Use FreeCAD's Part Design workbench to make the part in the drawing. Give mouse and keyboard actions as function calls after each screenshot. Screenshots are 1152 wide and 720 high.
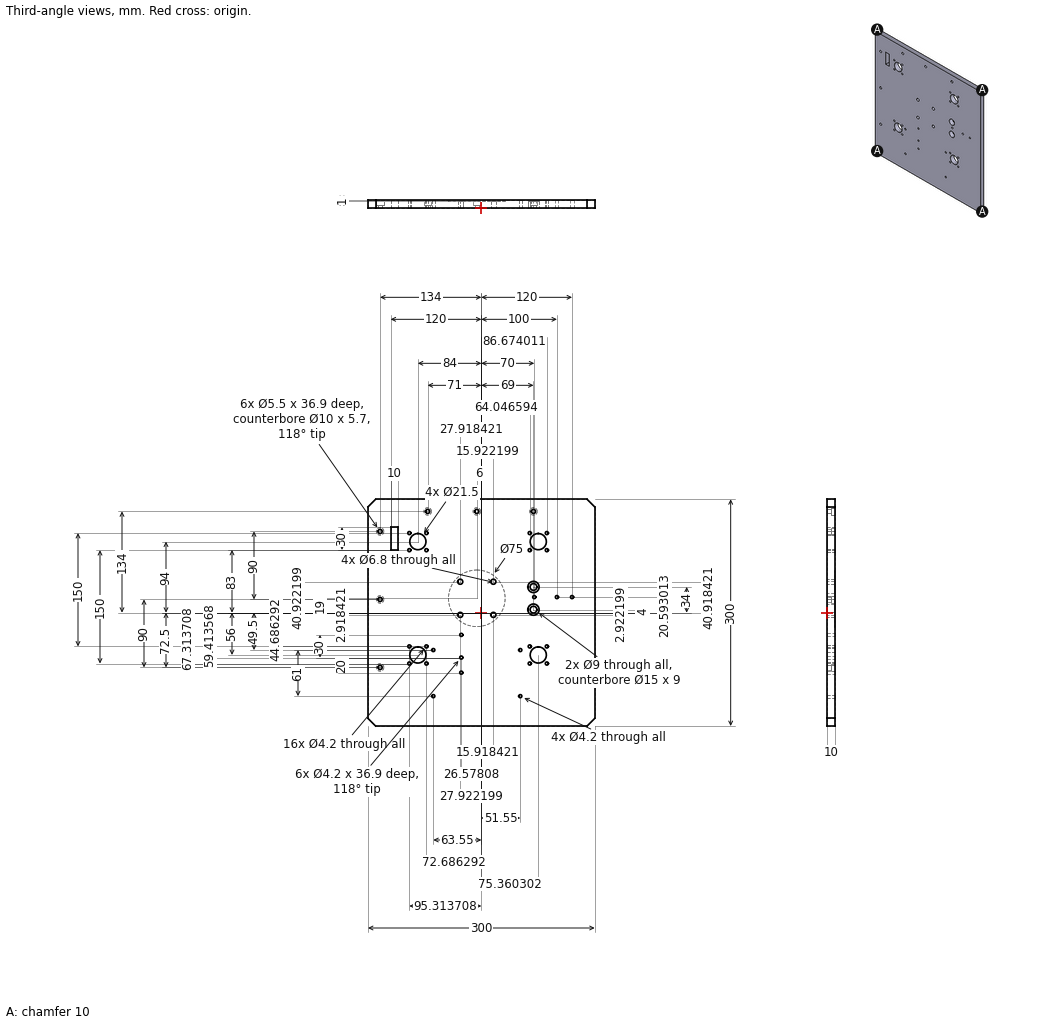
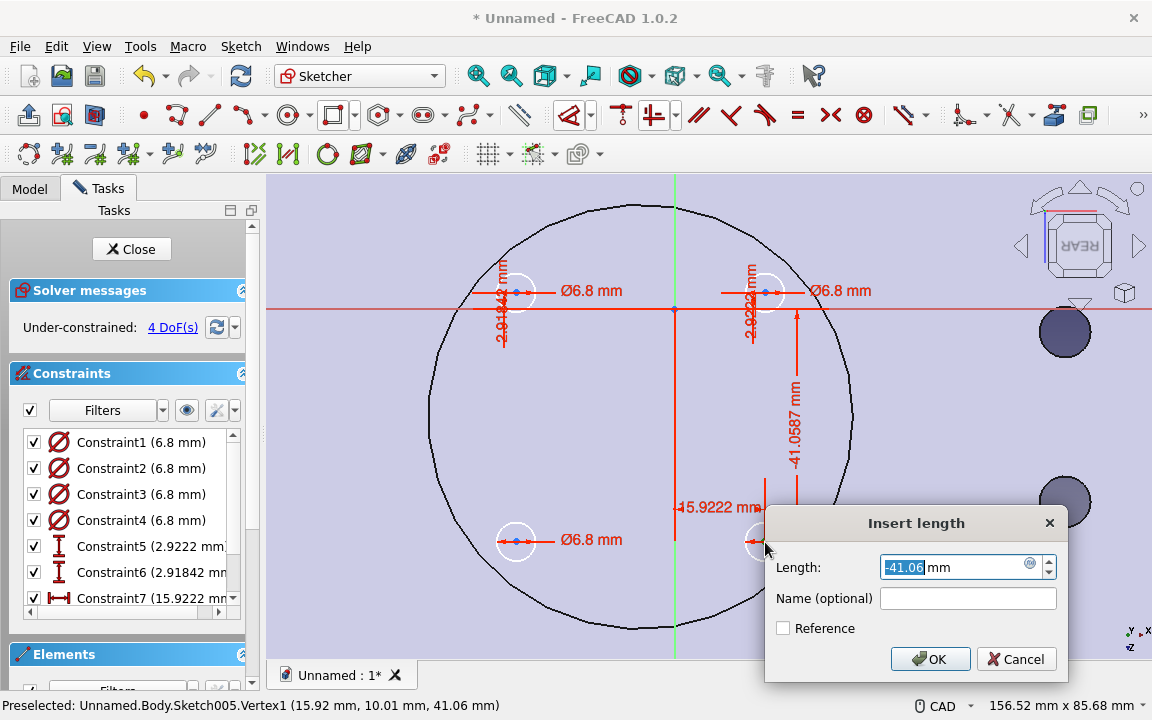
text(-40.918421)
key(Return)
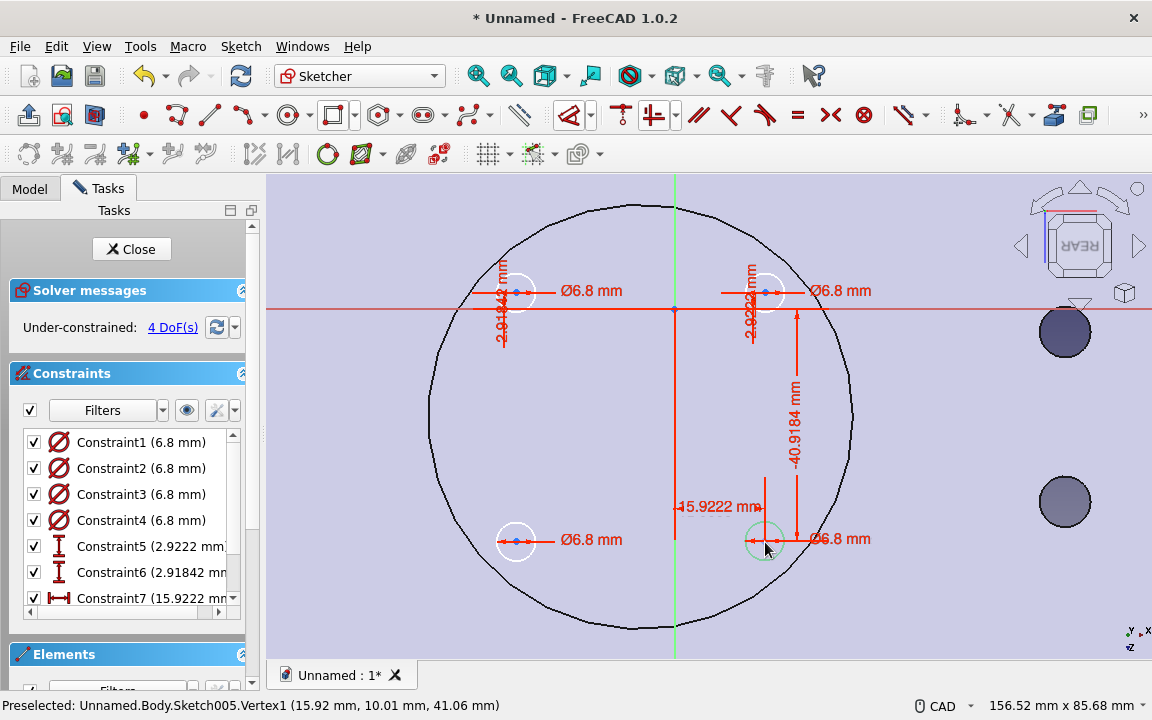
click(765, 293)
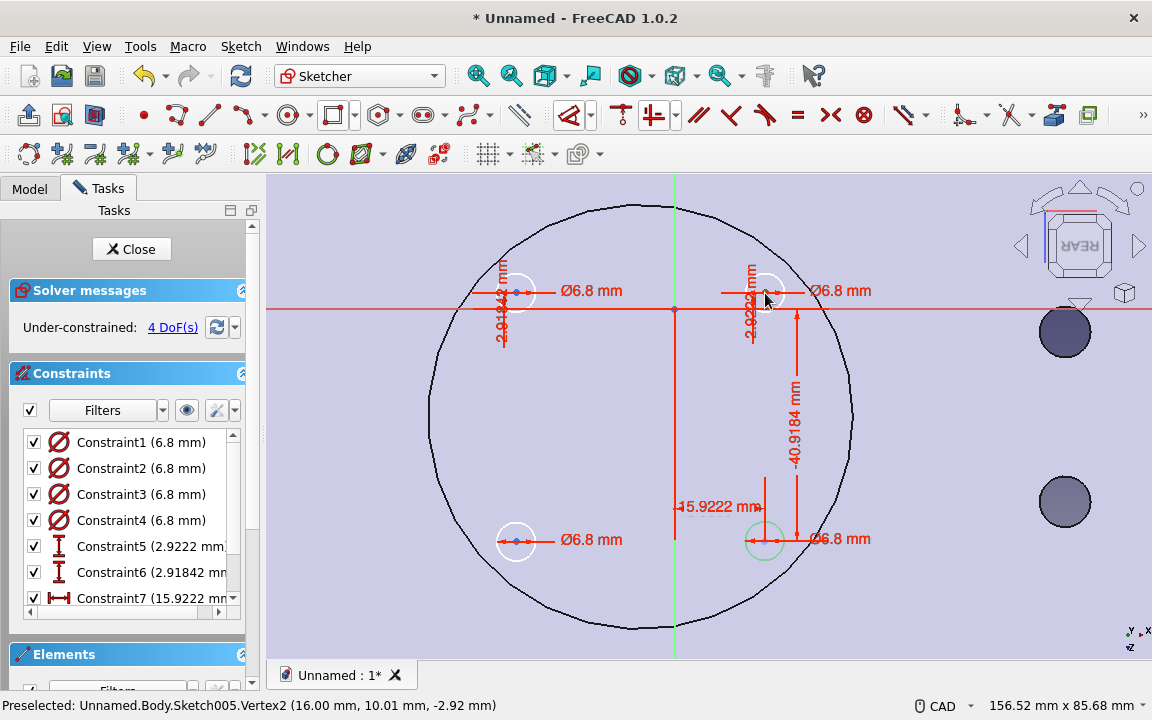
click(590, 116)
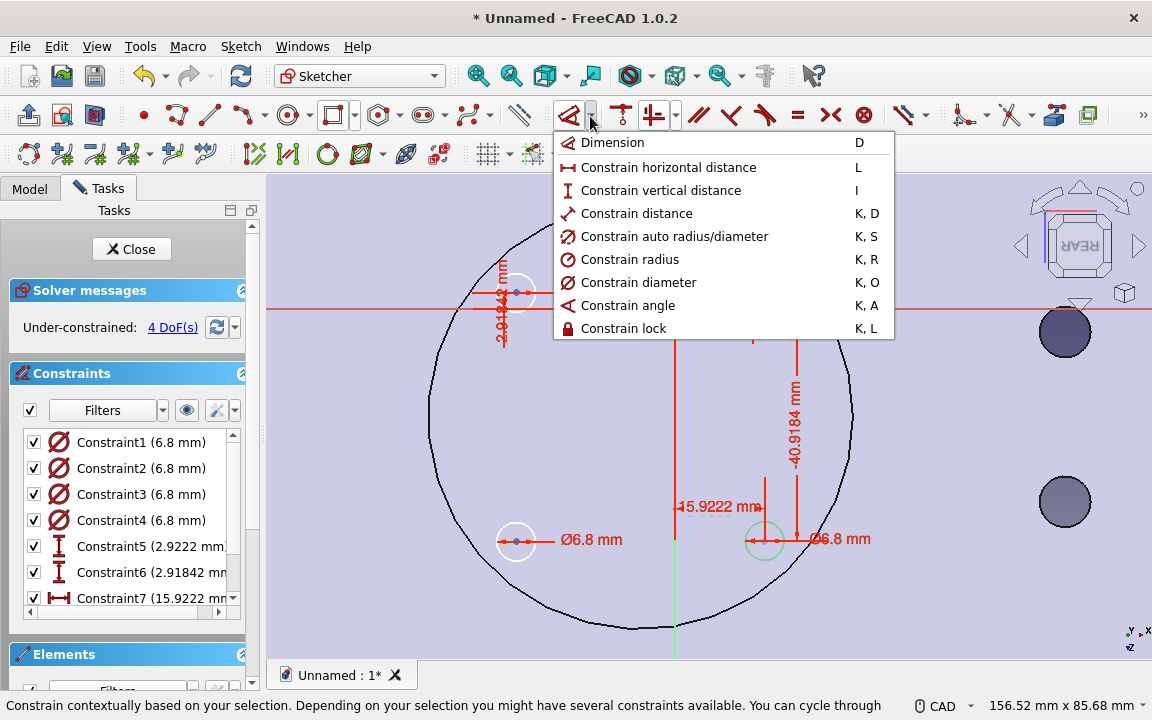
click(724, 168)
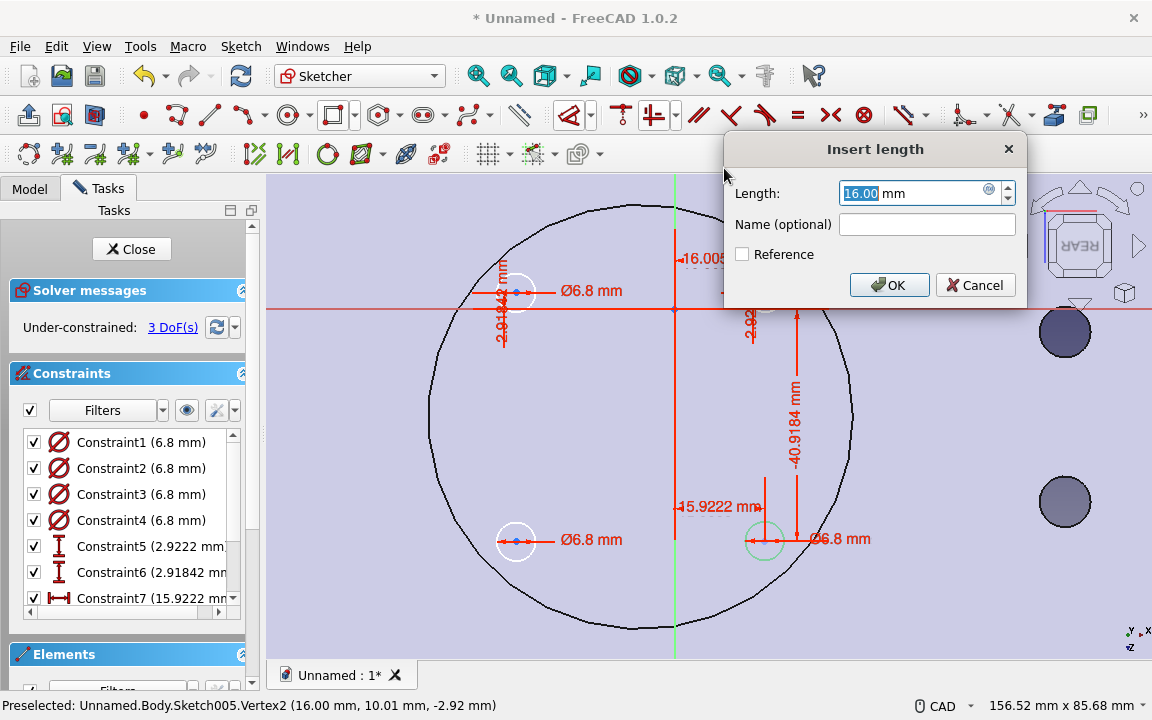
text(15.918421)
key(Return)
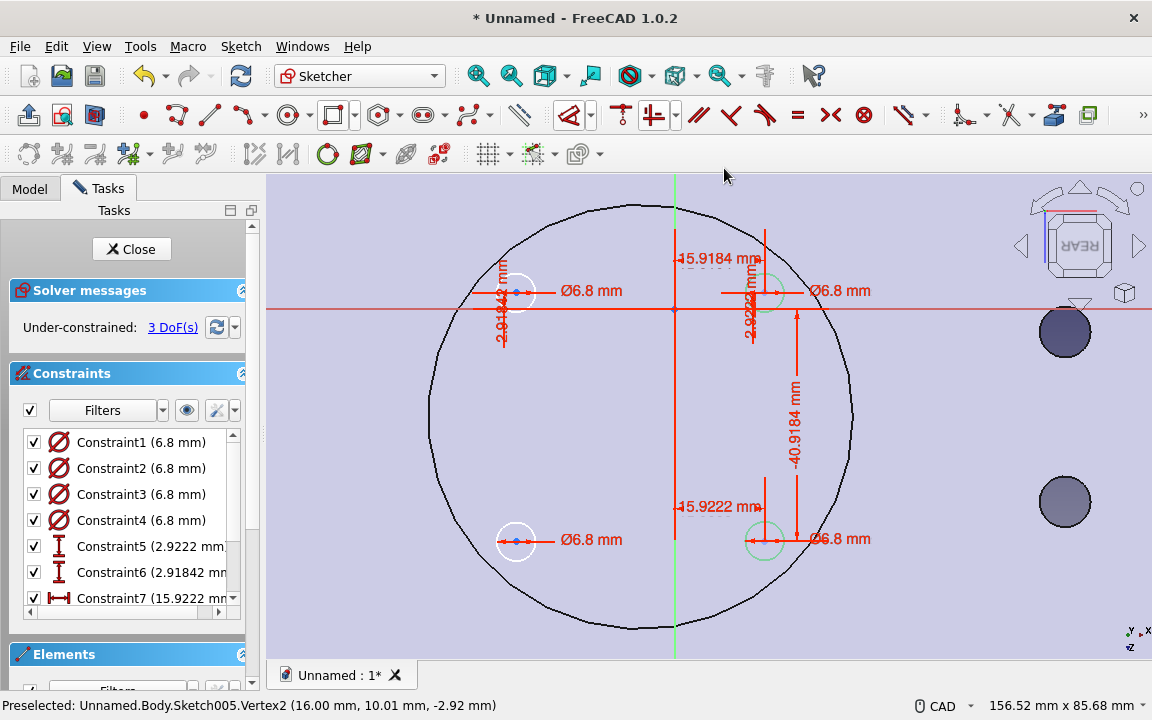
click(516, 293)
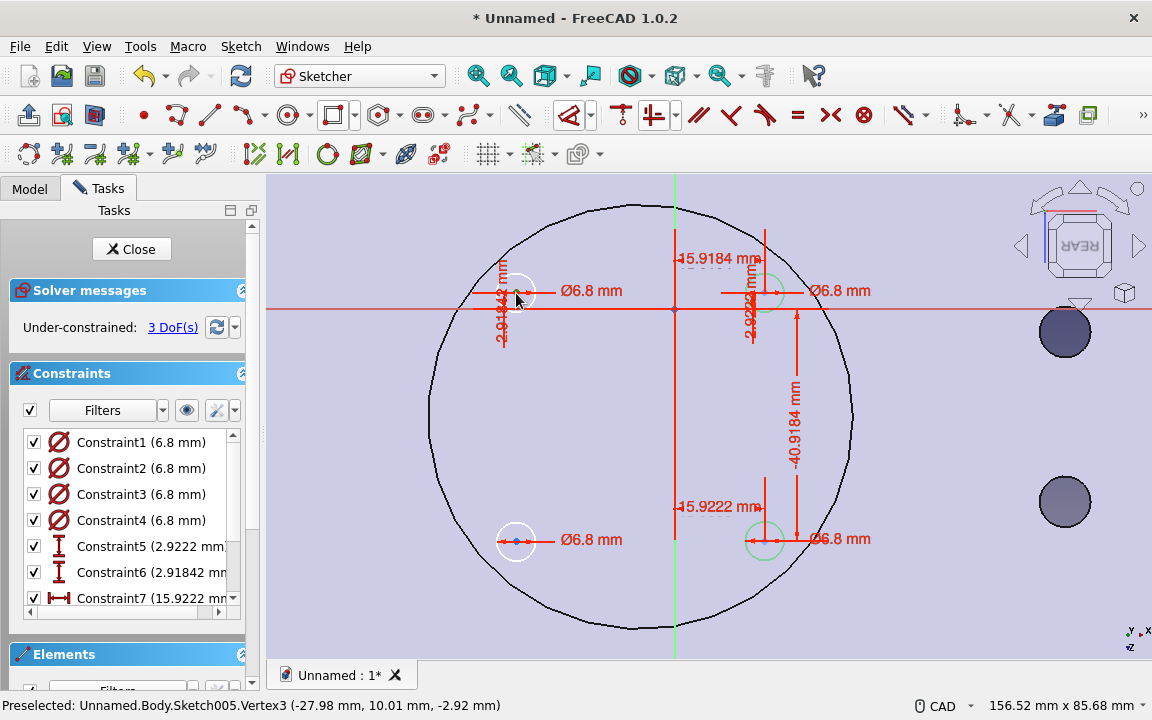
key(l)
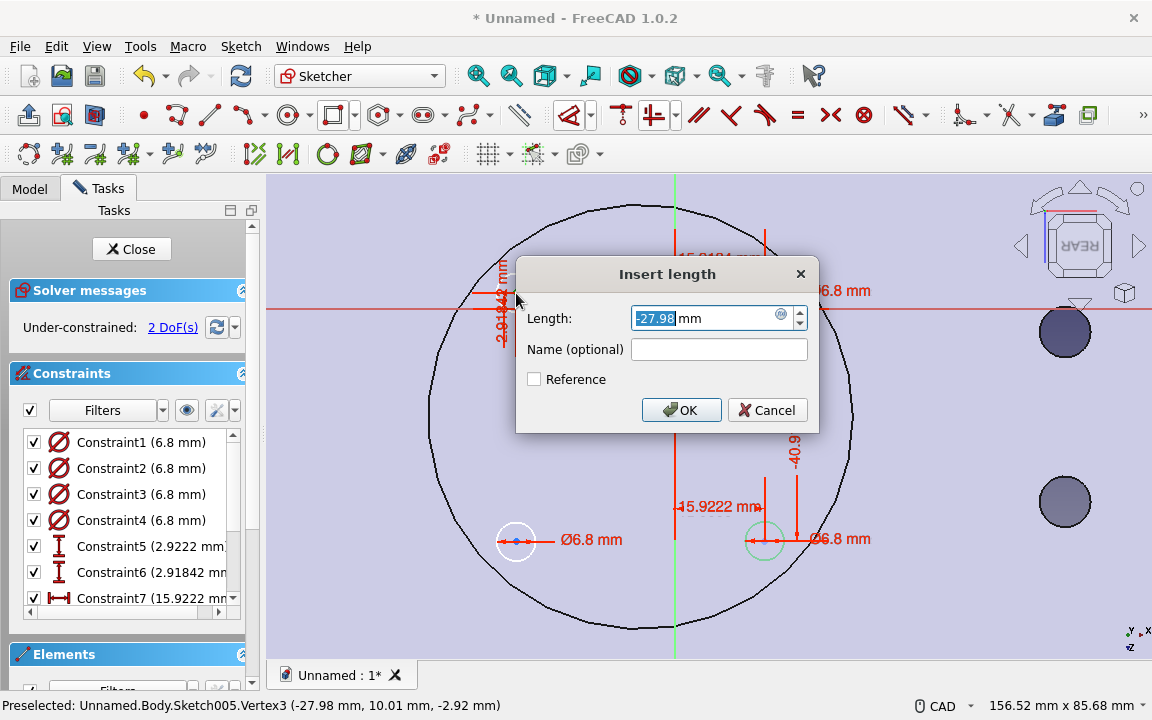
text(-27.922199)
key(Return)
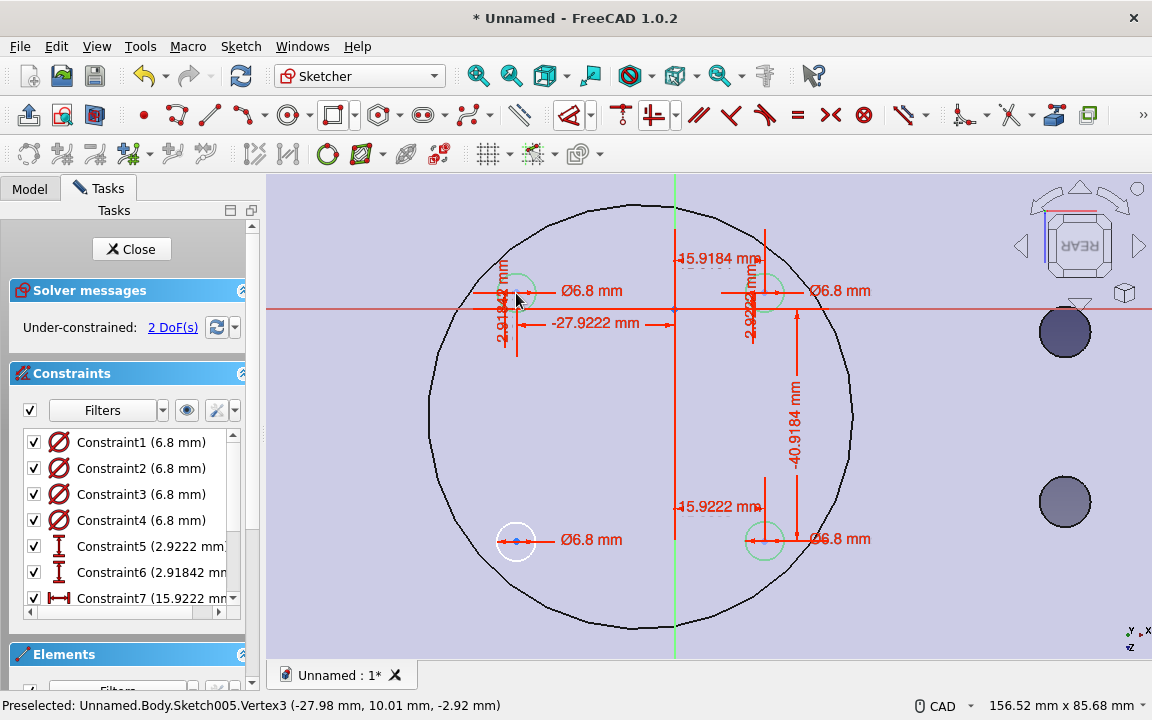
click(516, 542)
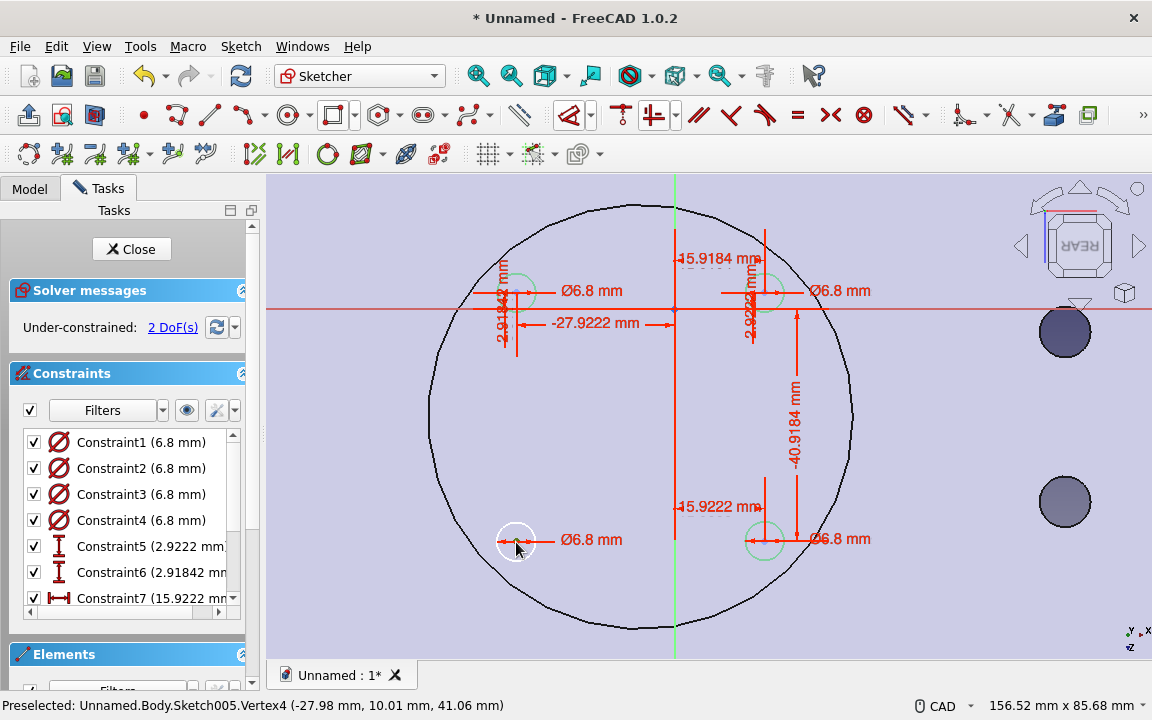
click(590, 116)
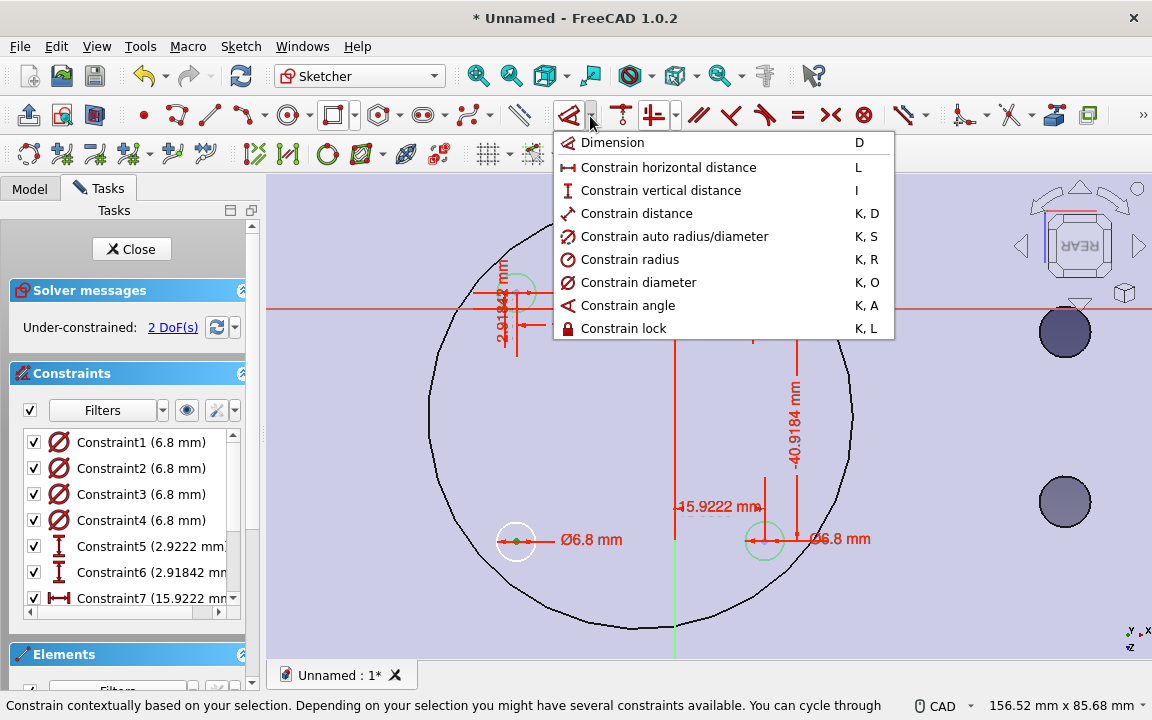
click(724, 168)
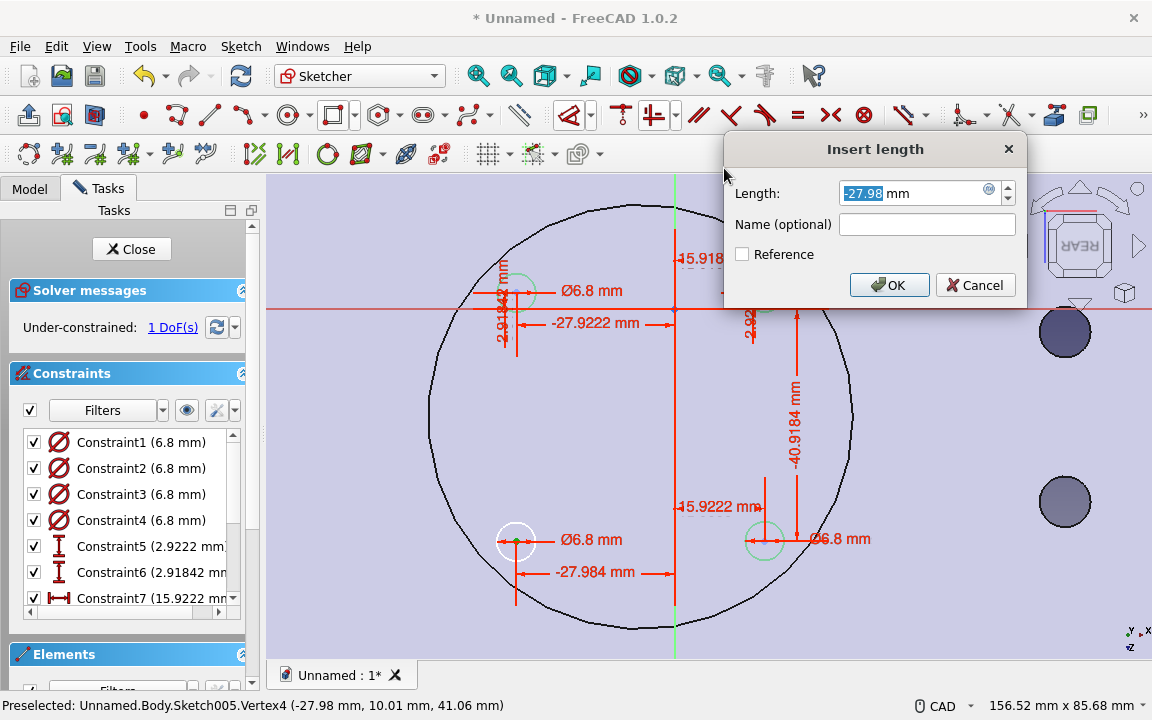
text(-27.918421)
key(Return)